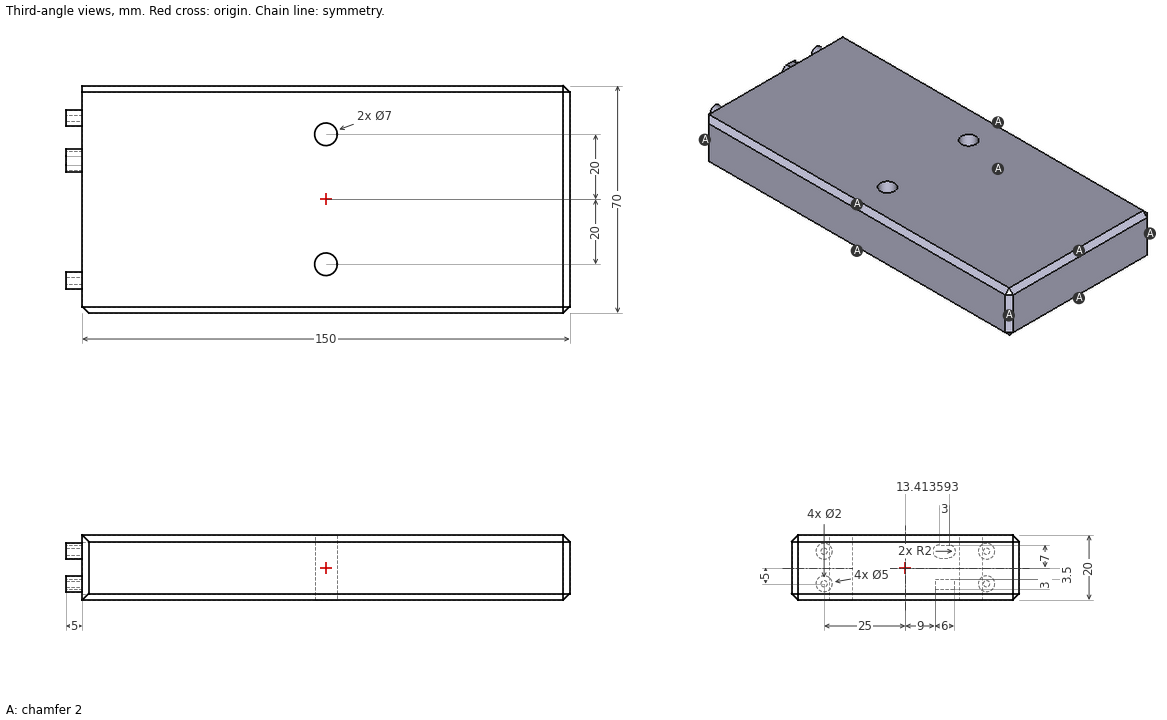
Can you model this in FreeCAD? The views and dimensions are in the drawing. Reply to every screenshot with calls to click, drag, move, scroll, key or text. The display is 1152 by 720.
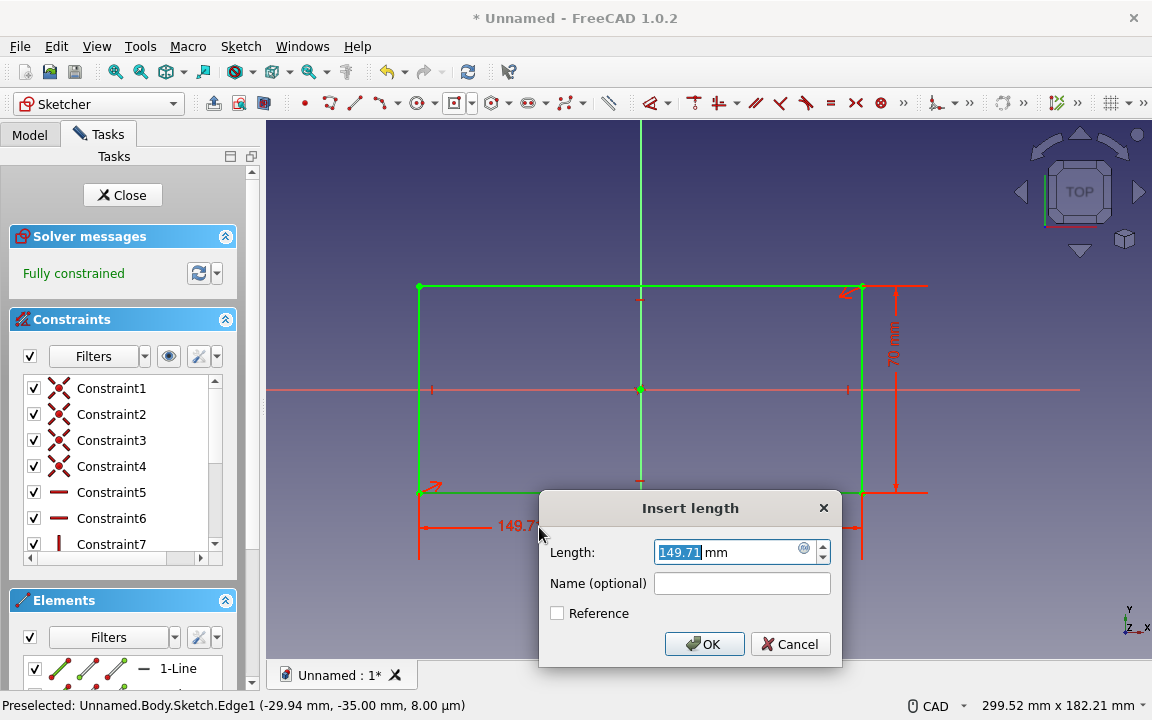
text(150)
key(Return)
key(Escape)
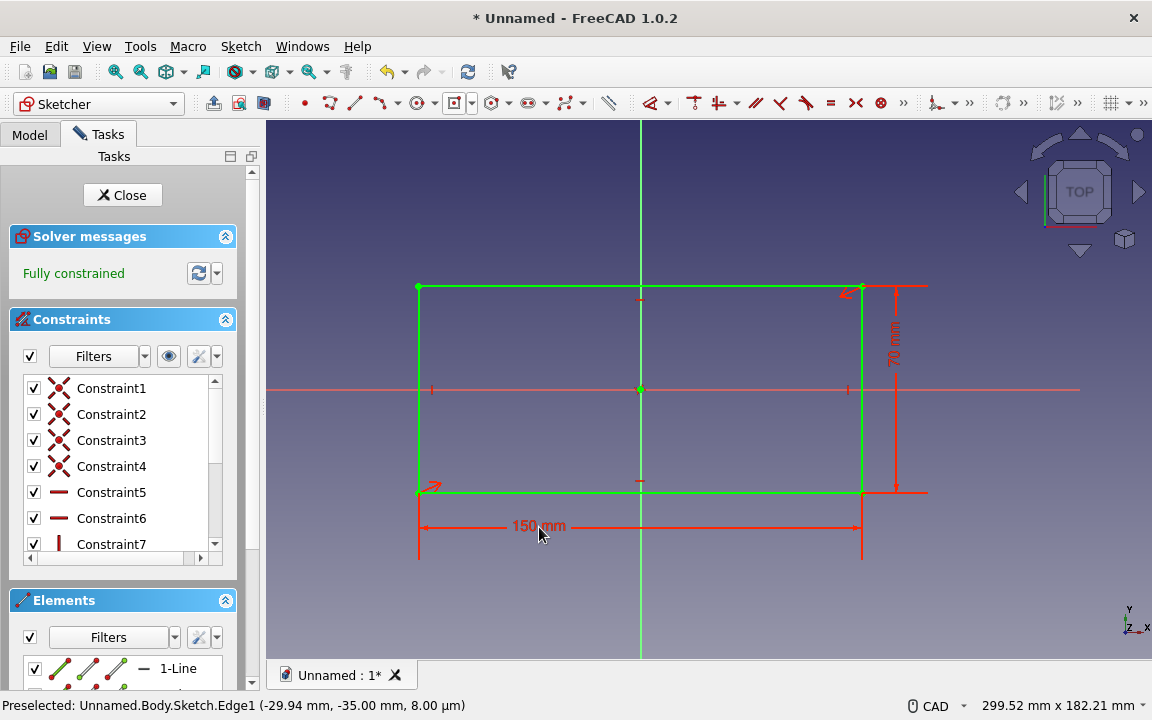
click(123, 195)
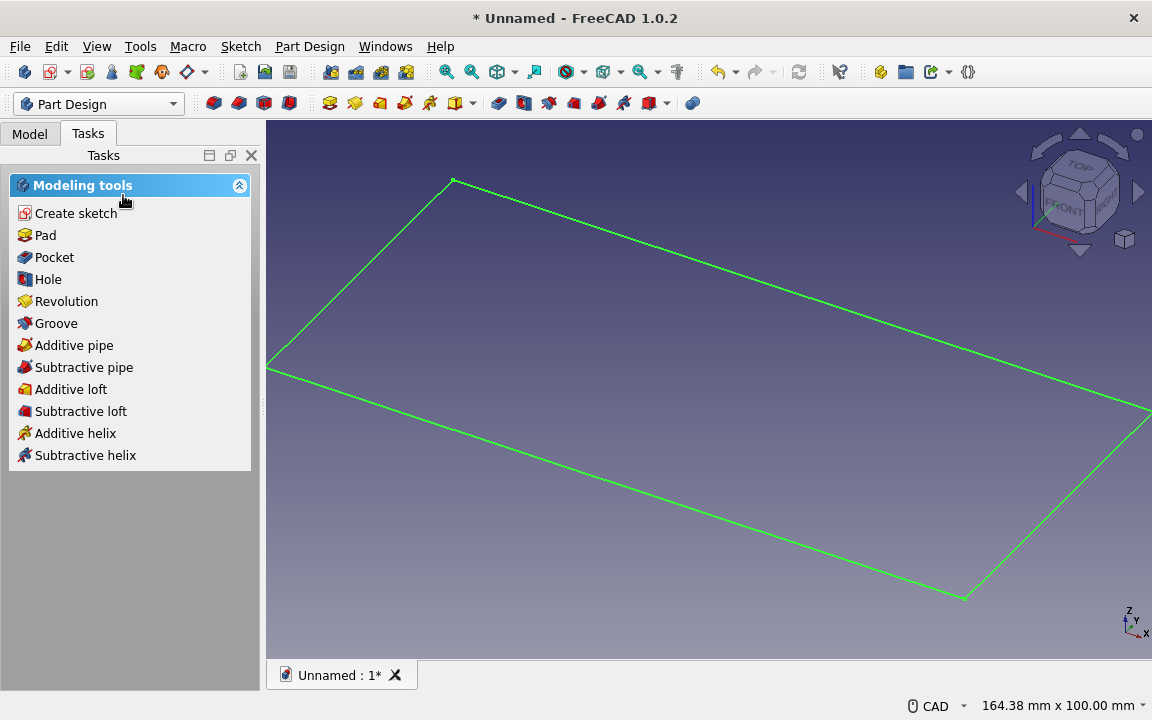
click(330, 104)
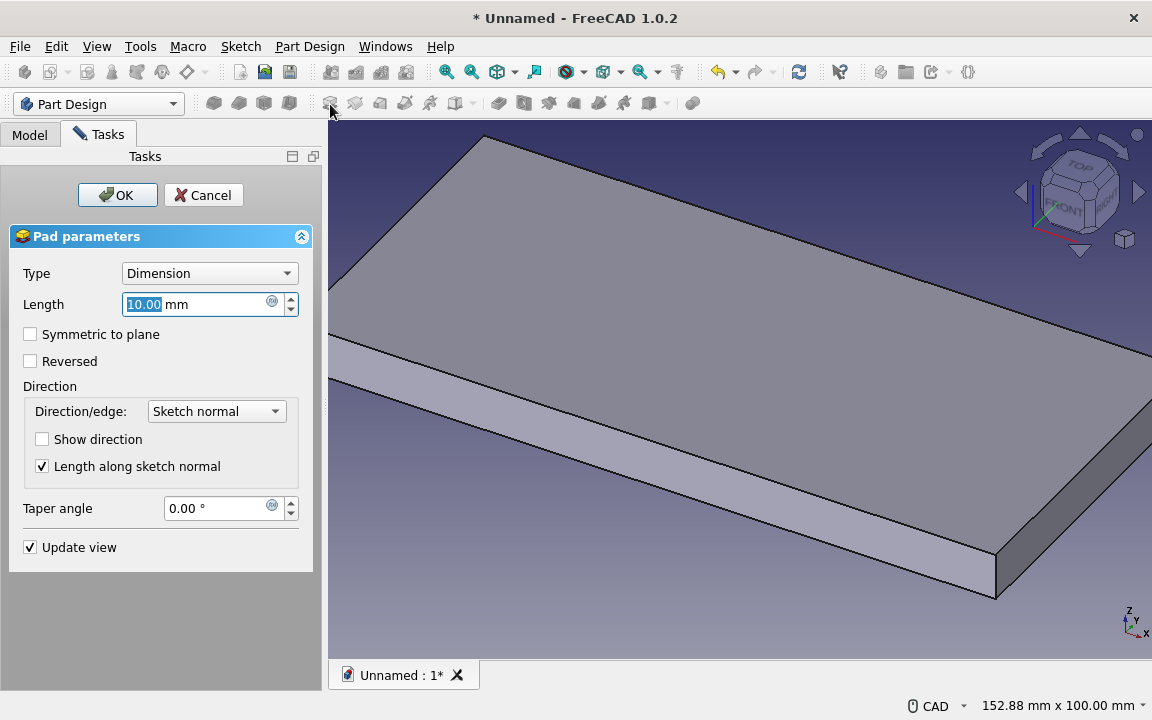
text(20)
key(Tab)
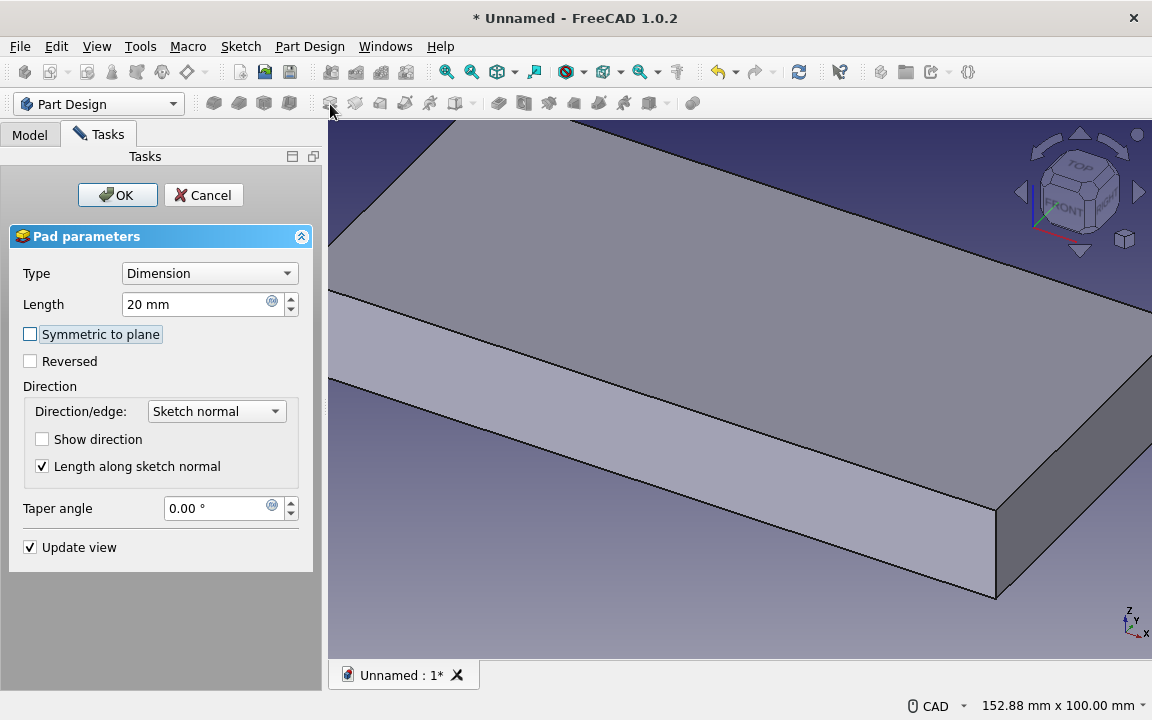
click(31, 334)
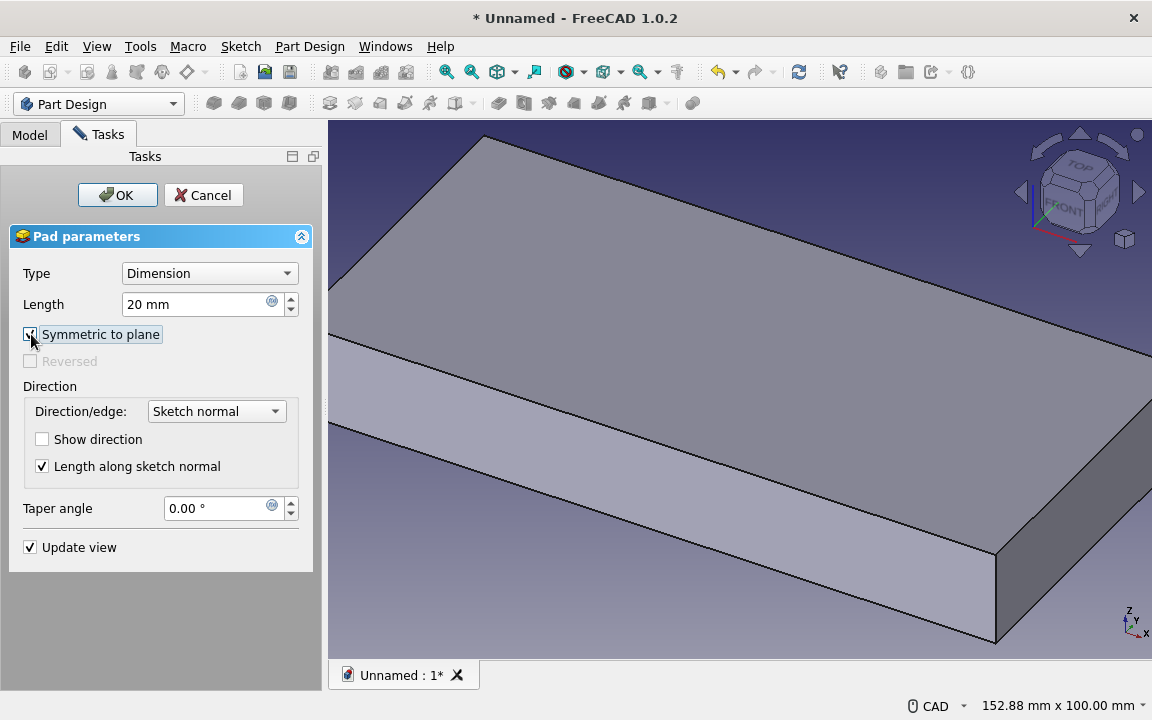
click(118, 195)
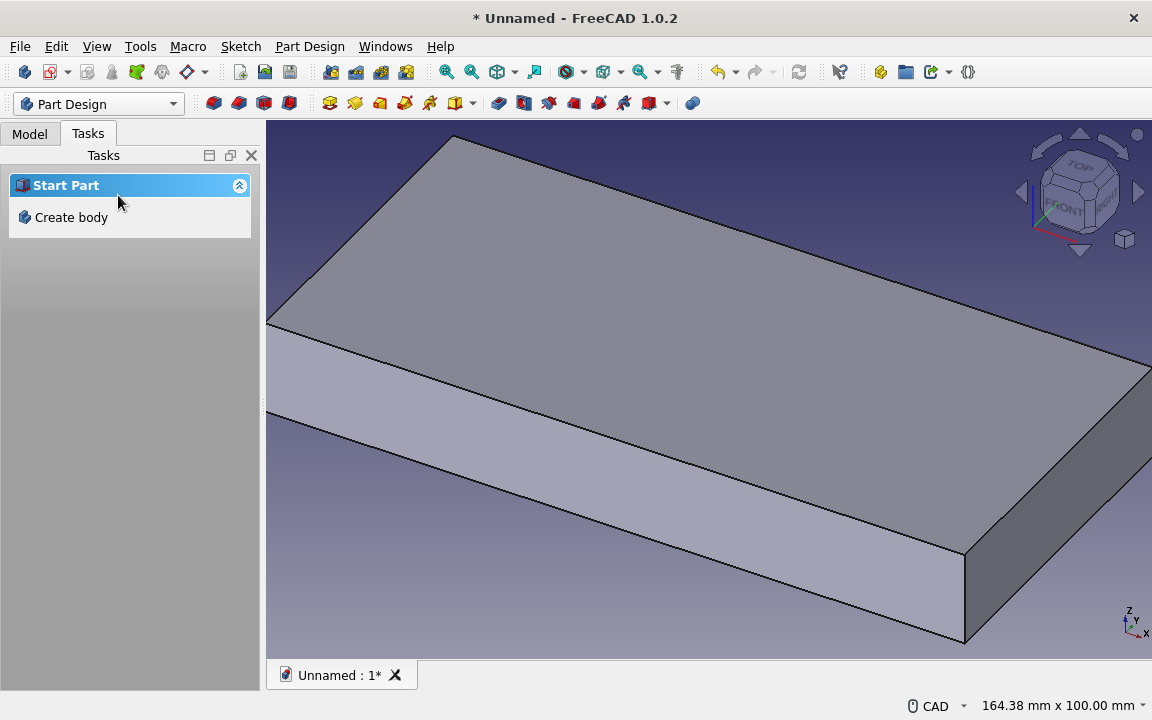
click(447, 72)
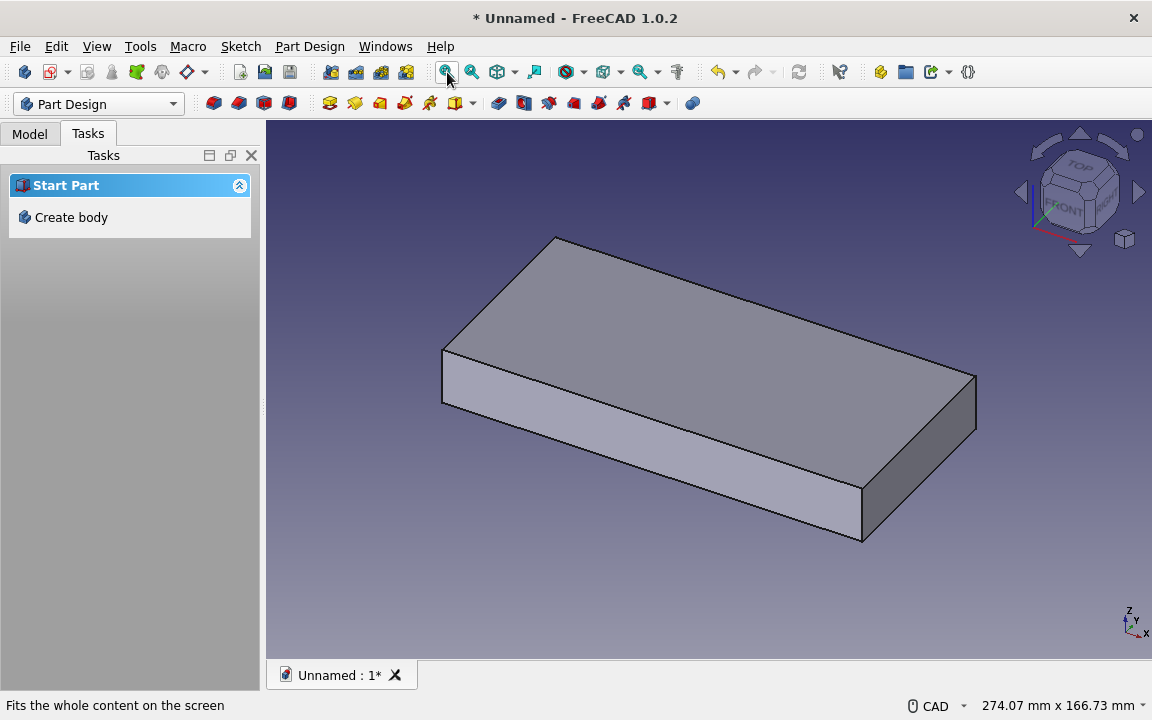
key(6)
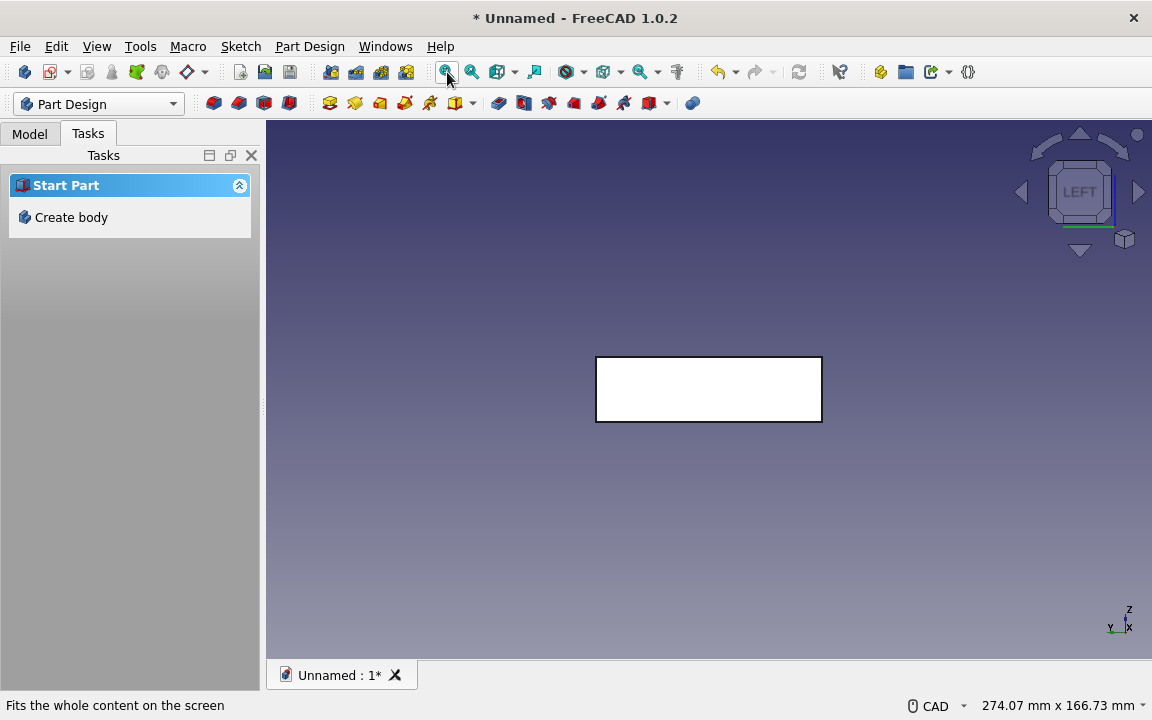
click(447, 72)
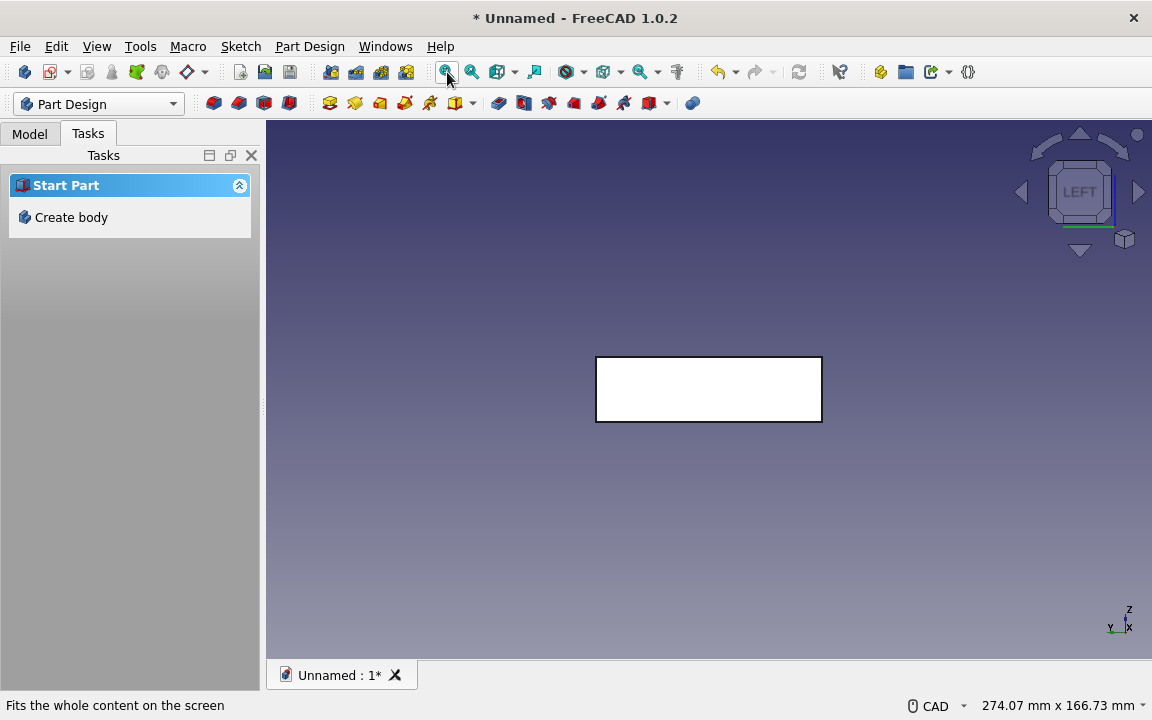
click(644, 388)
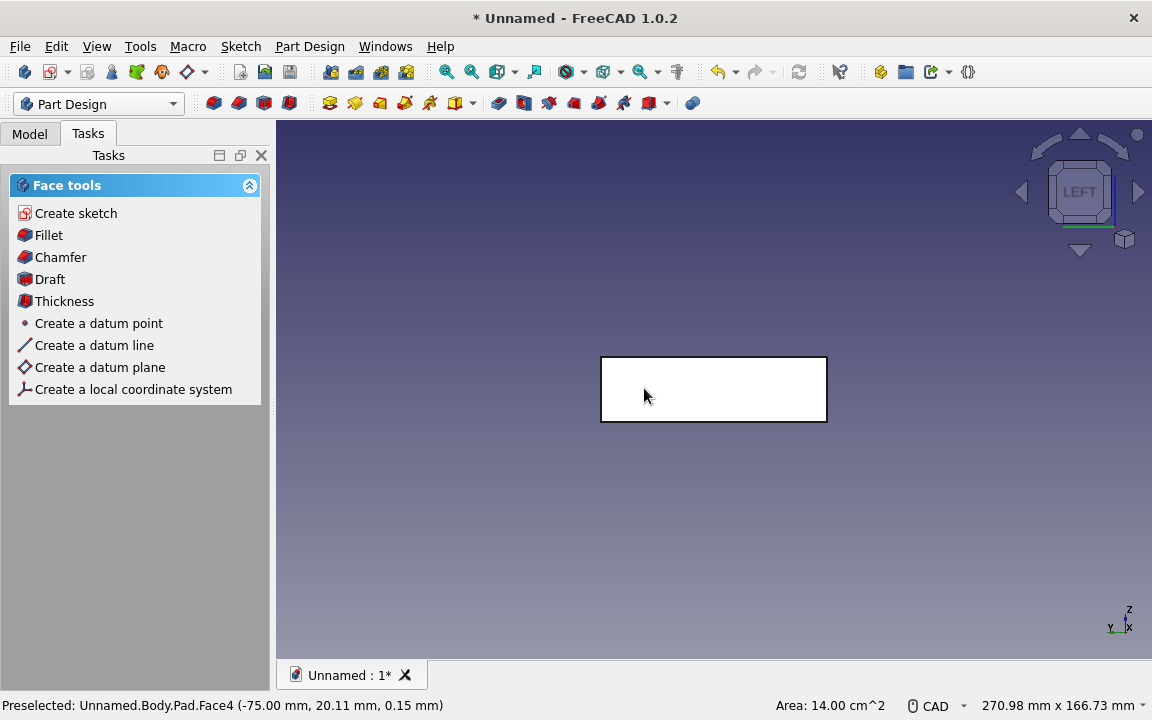
click(50, 72)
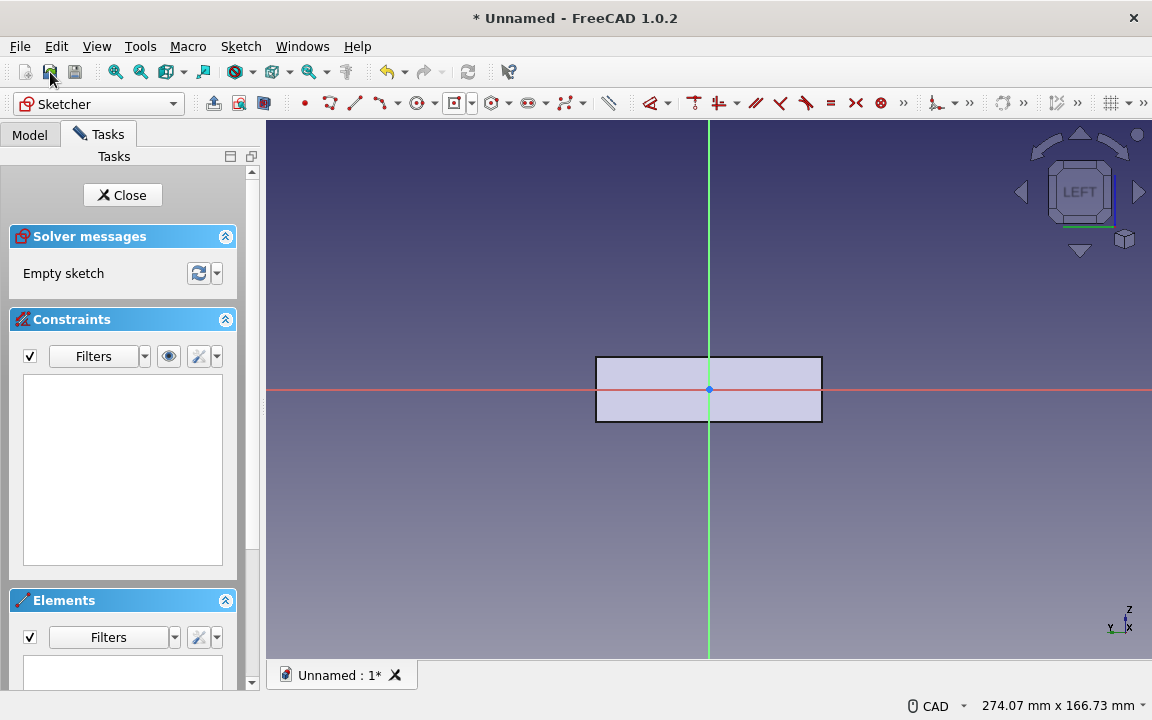
scroll(749, 390, up, 5)